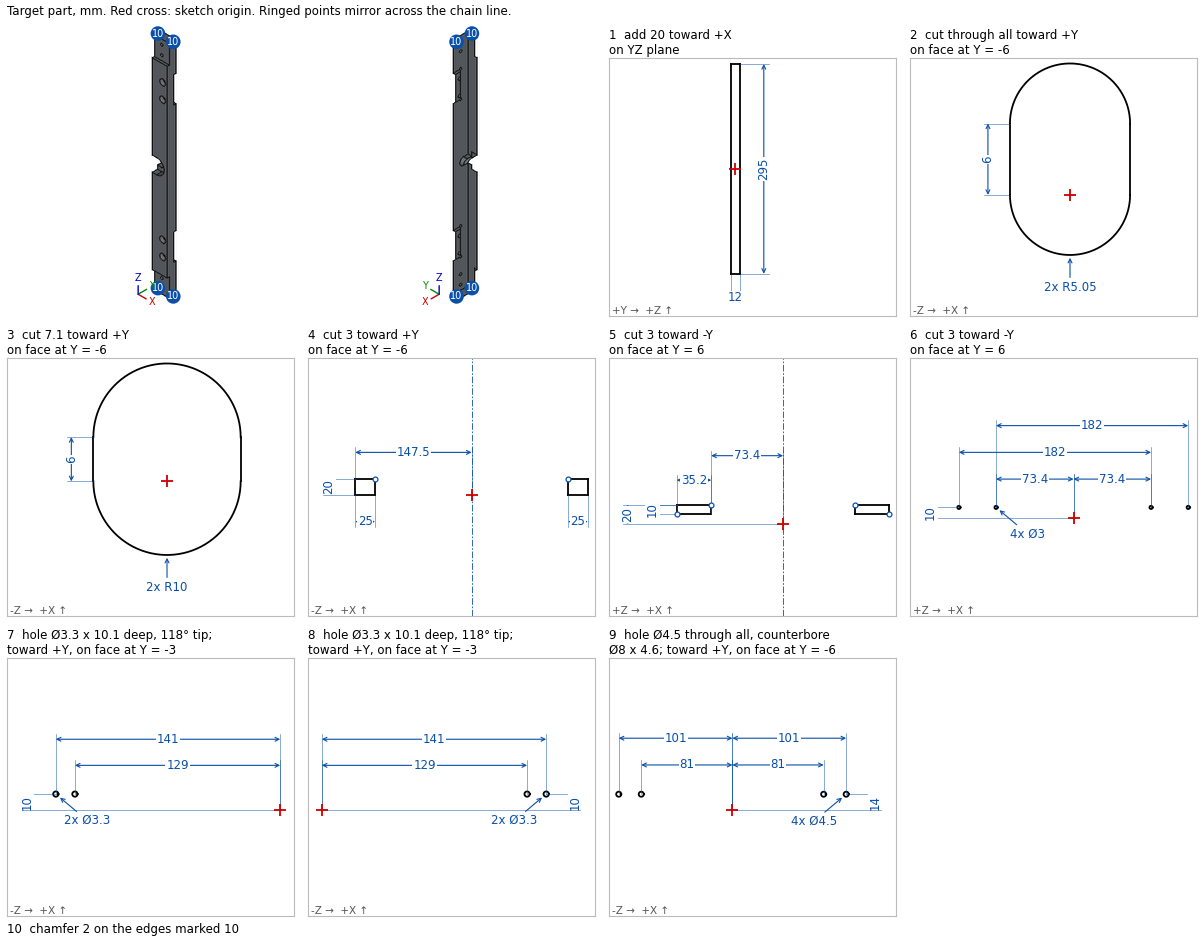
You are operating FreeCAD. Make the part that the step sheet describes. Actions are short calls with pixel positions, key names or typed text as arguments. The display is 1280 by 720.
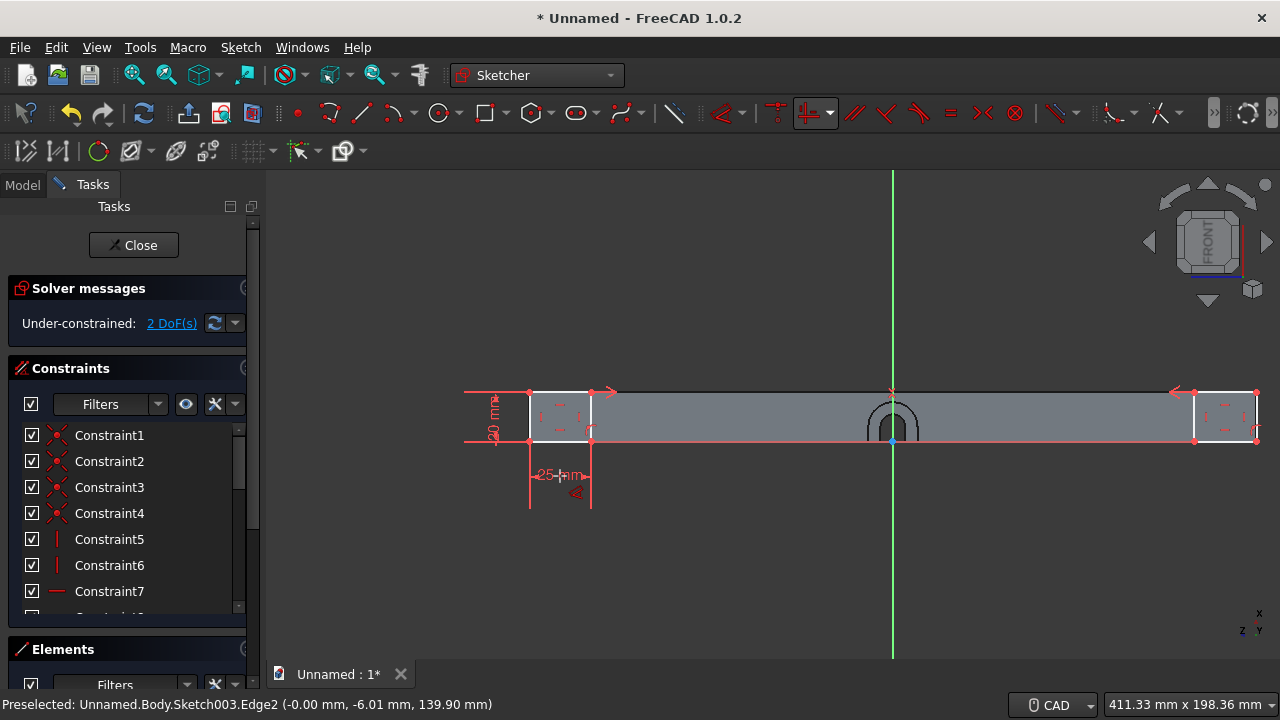
scroll(294, 403, down, 1)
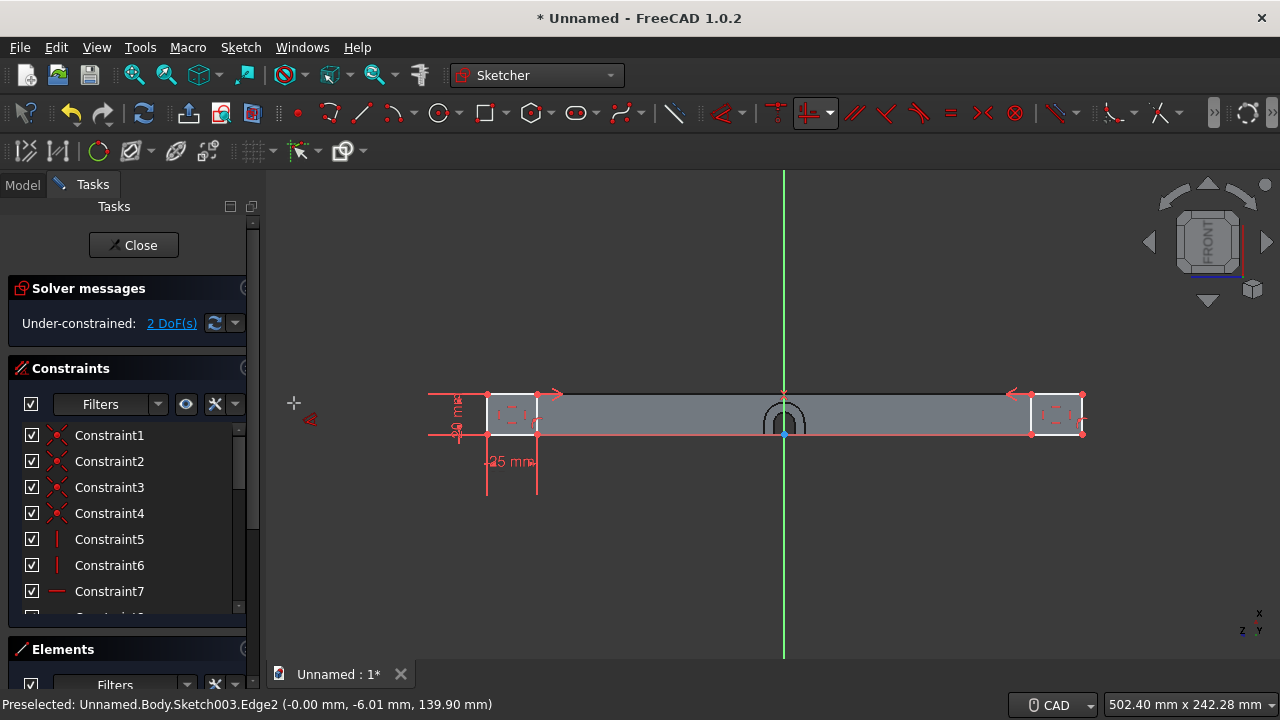
click(1047, 435)
click(1057, 469)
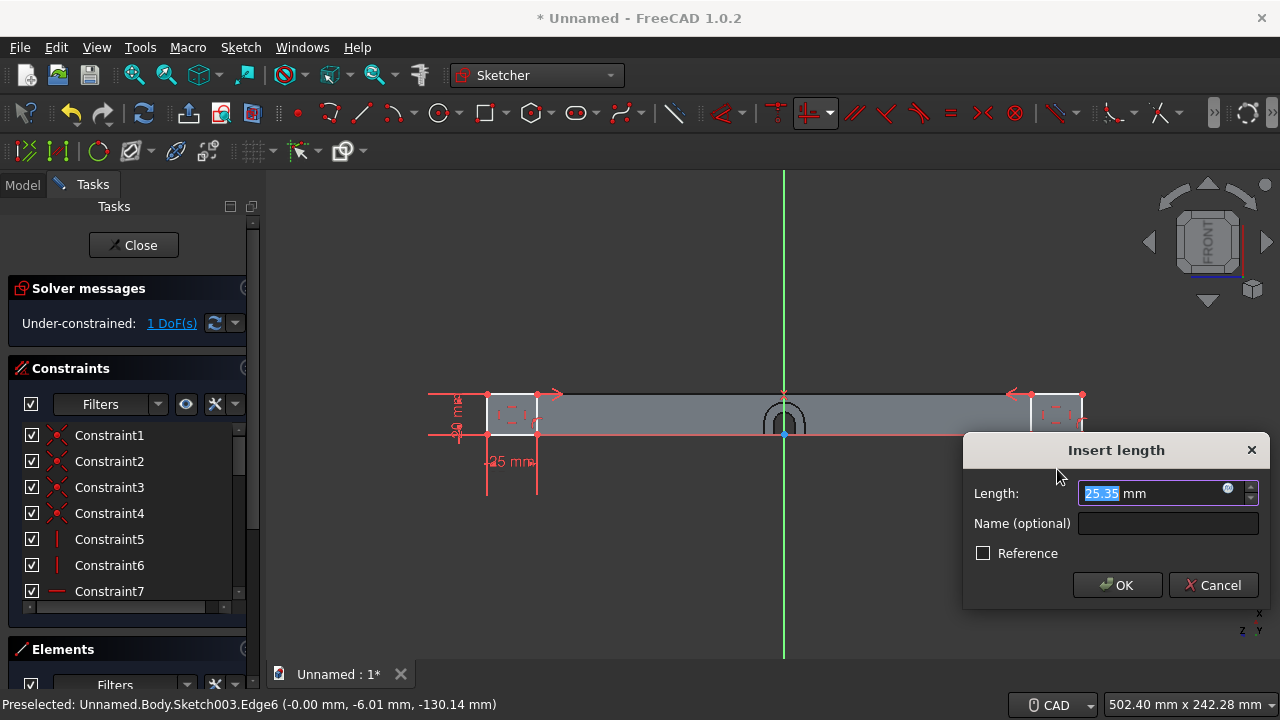
text(25)
key(Return)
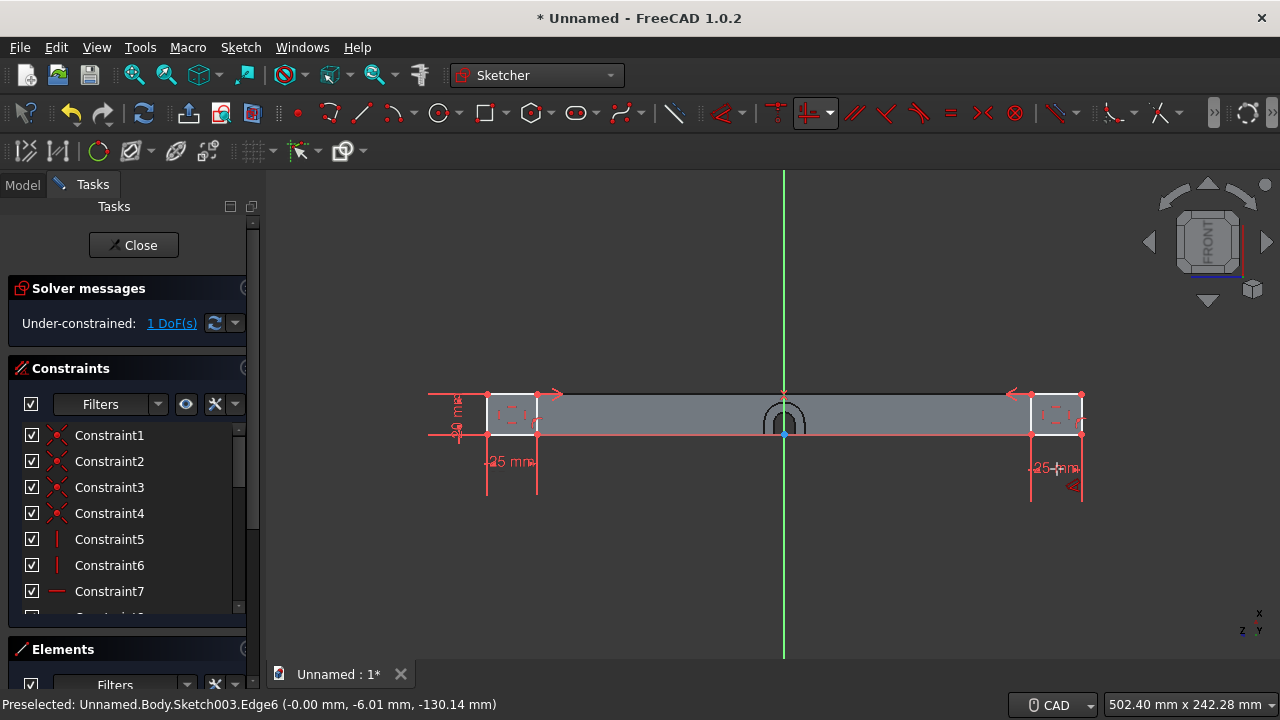
click(487, 394)
click(636, 469)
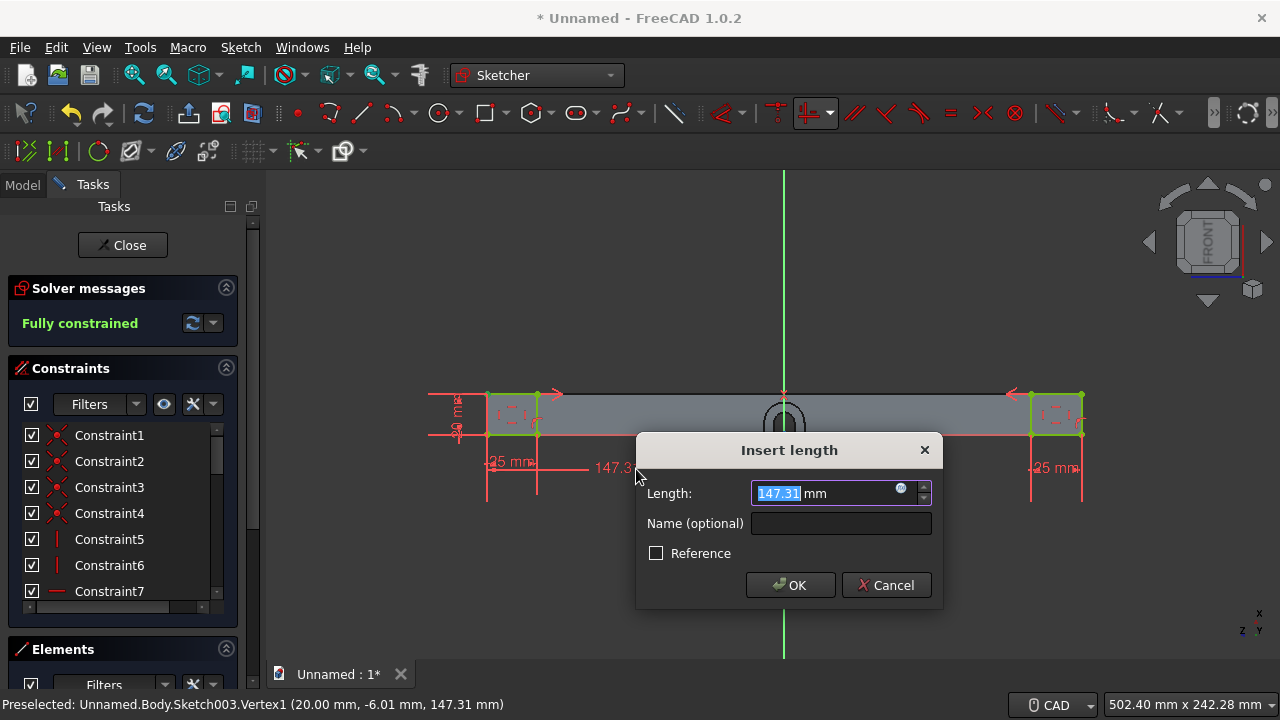
text(147.5)
key(Return)
key(Escape)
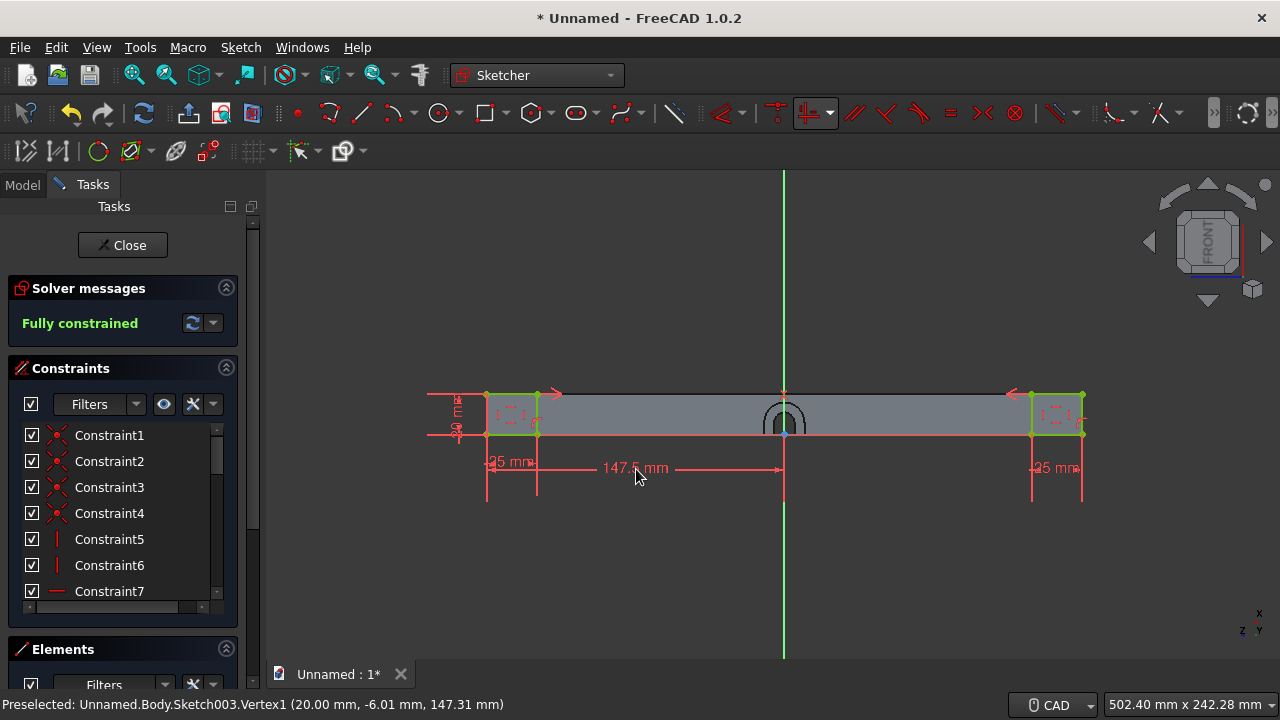
click(123, 245)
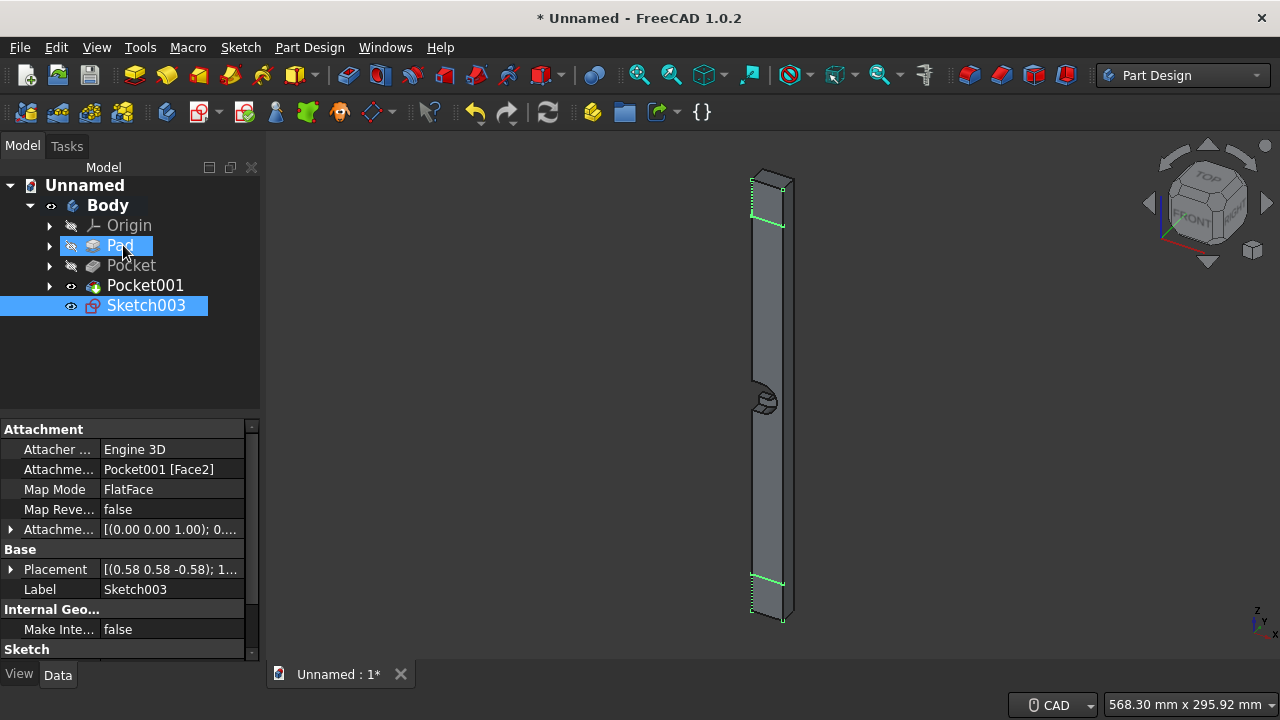
click(350, 76)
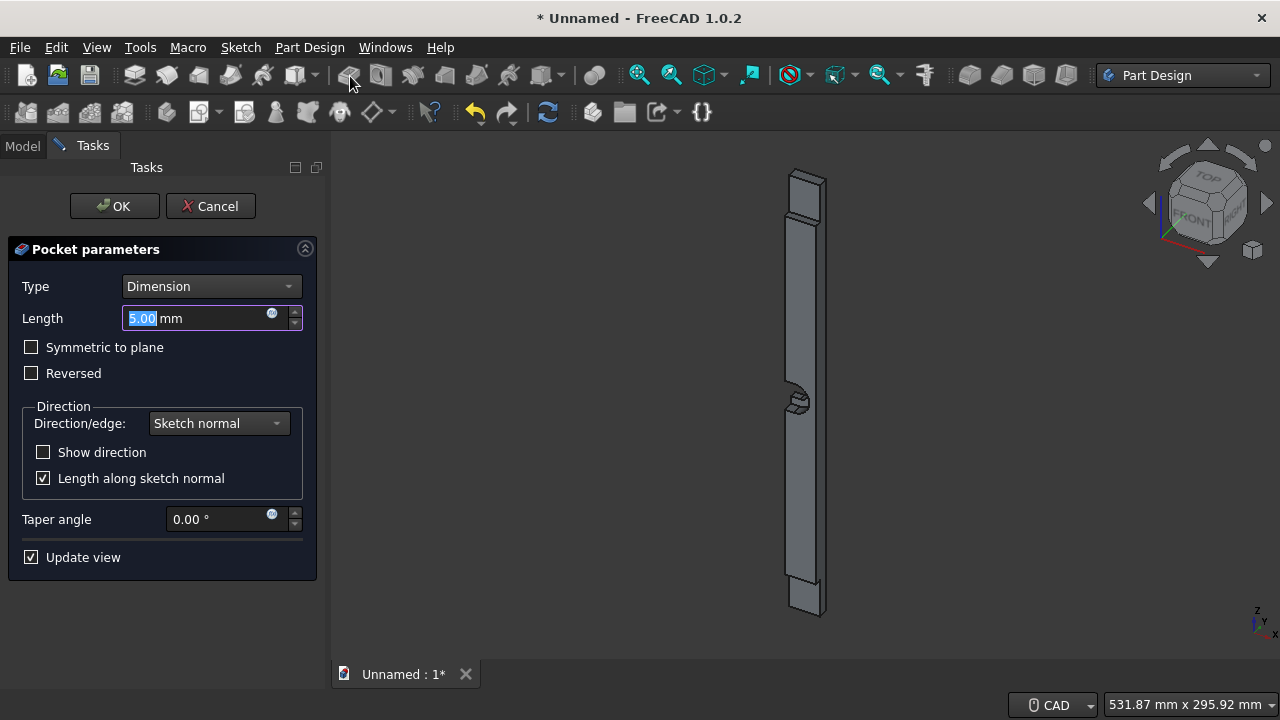
text(3)
key(Tab)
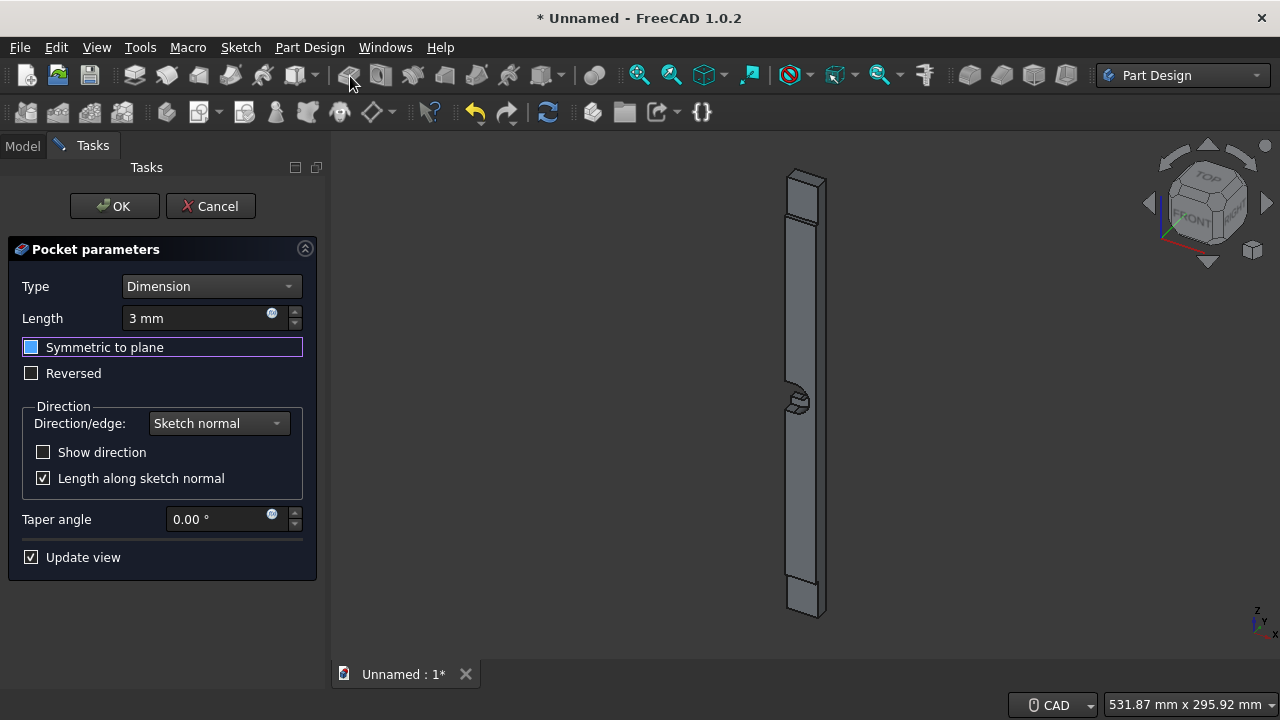
click(115, 206)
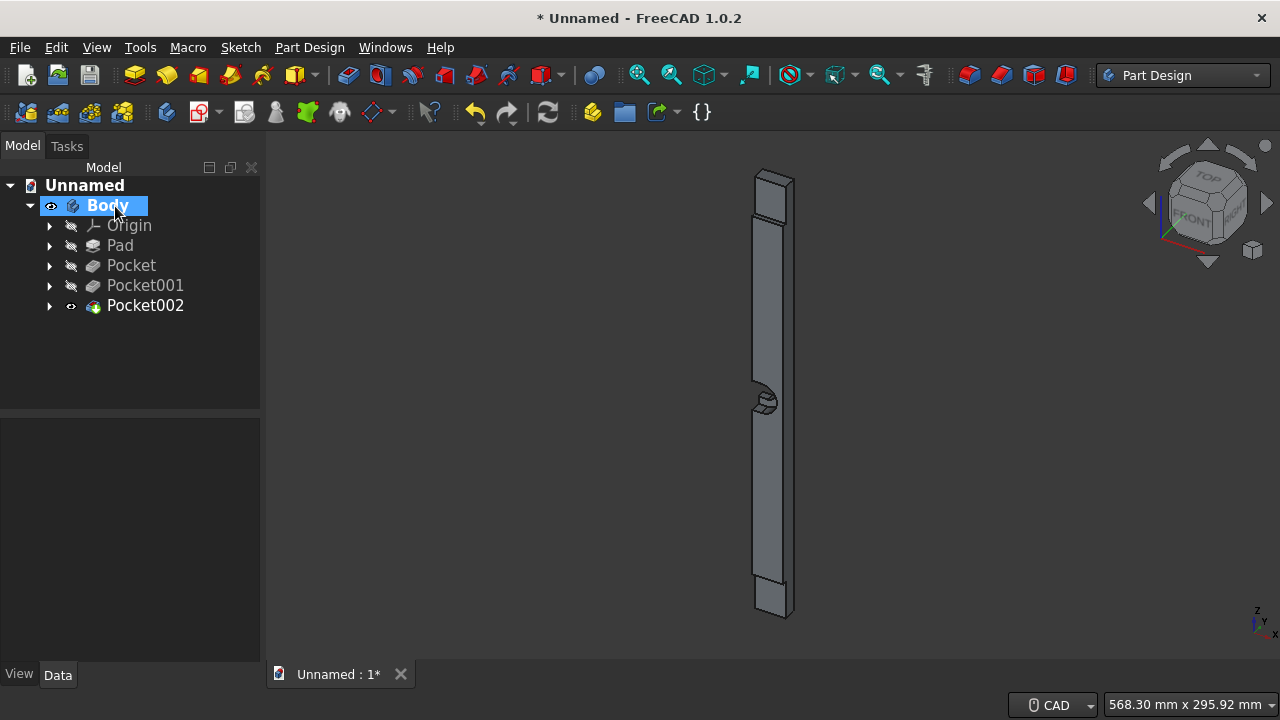
key(4)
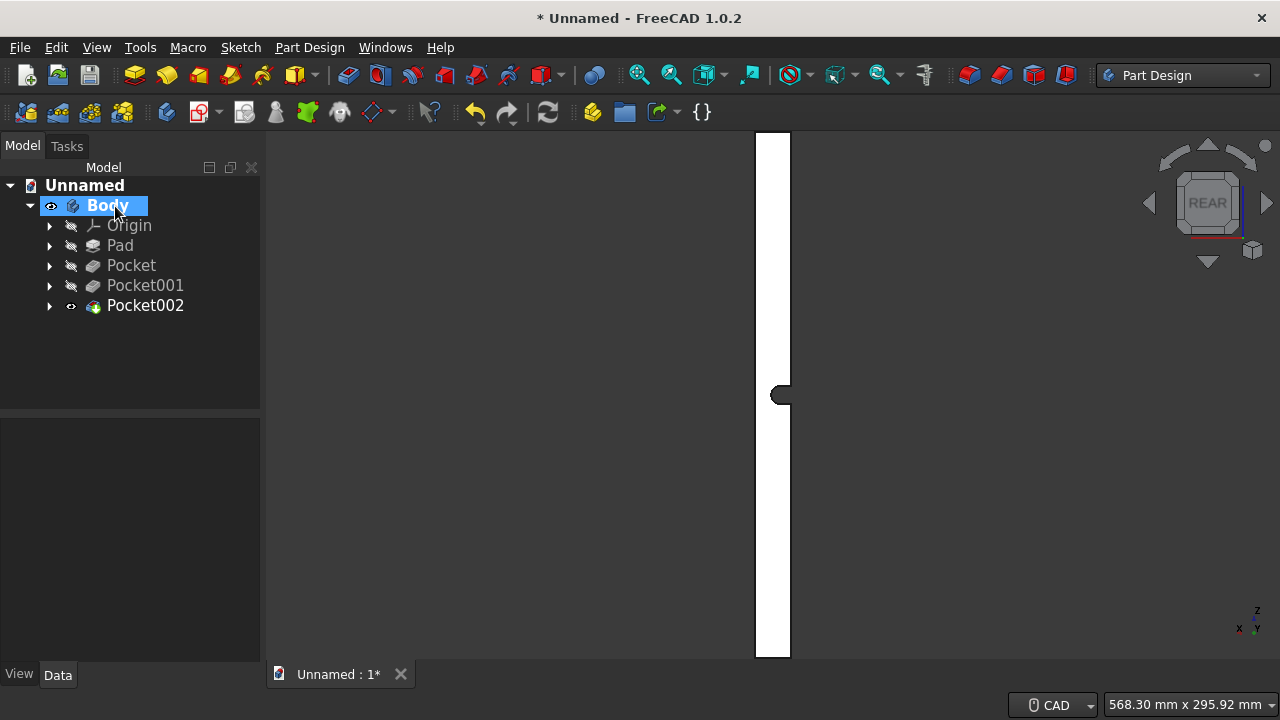
click(773, 319)